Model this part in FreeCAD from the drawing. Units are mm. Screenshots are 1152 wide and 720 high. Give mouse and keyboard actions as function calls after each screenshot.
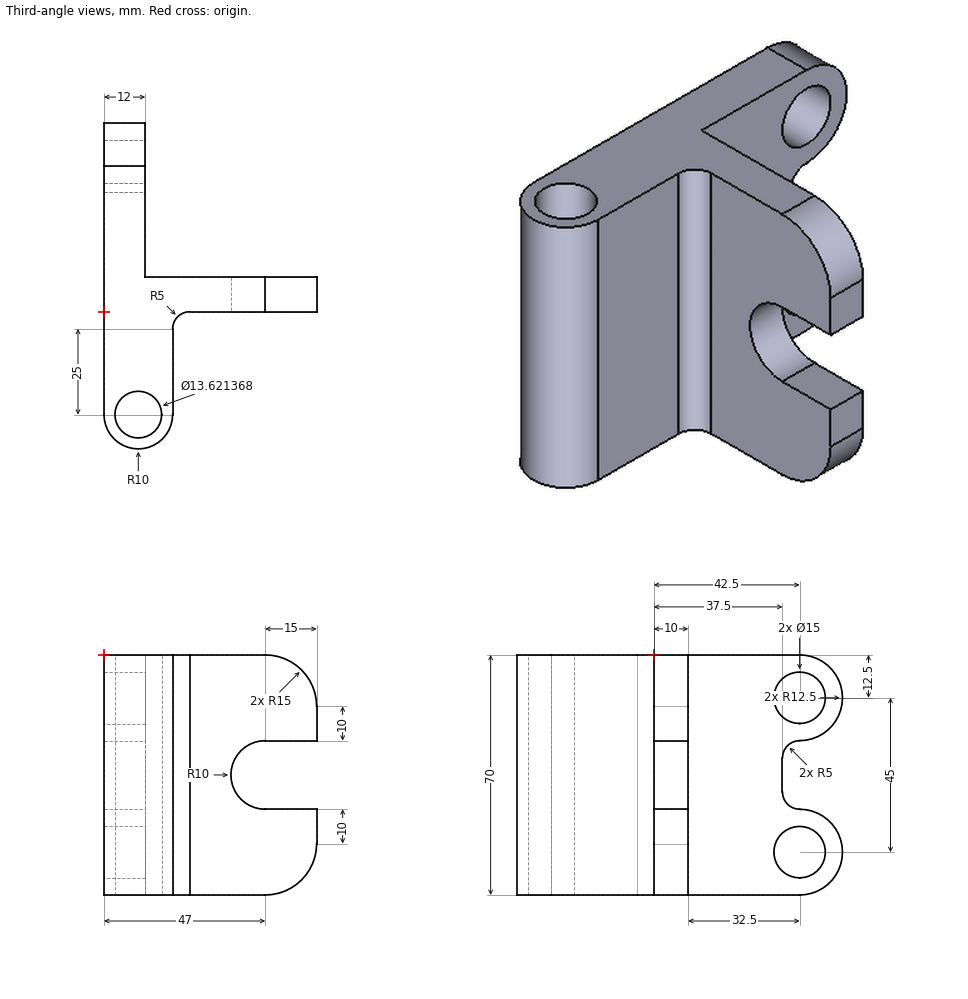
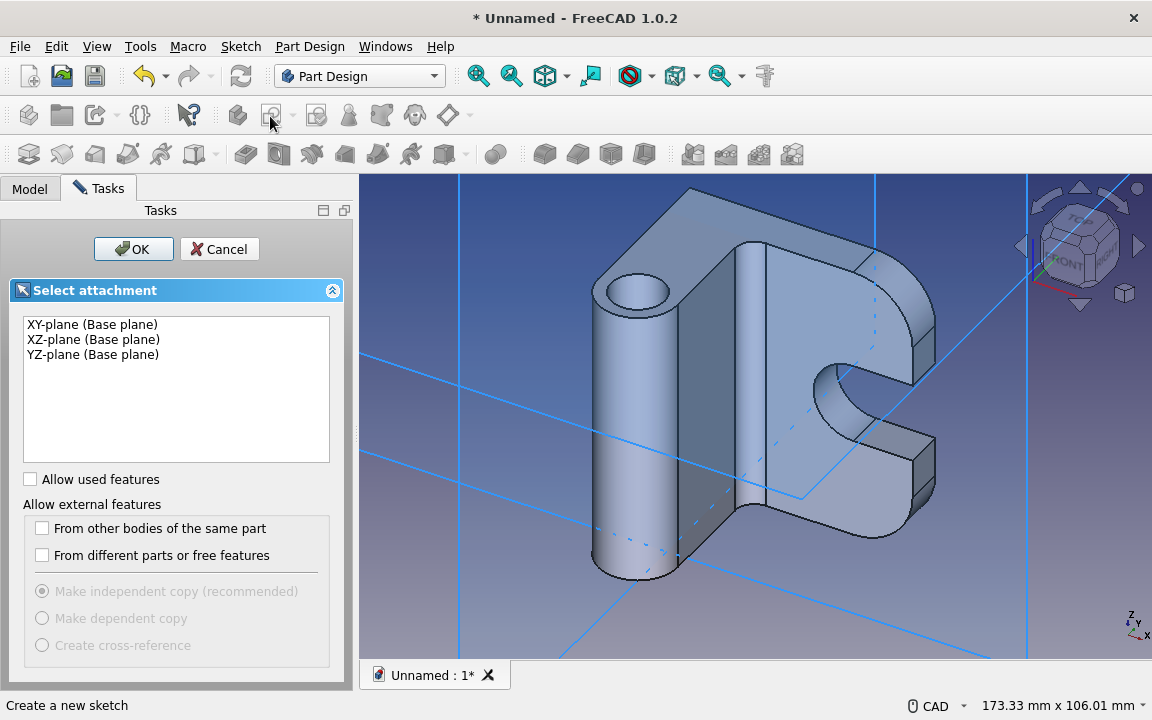
click(84, 354)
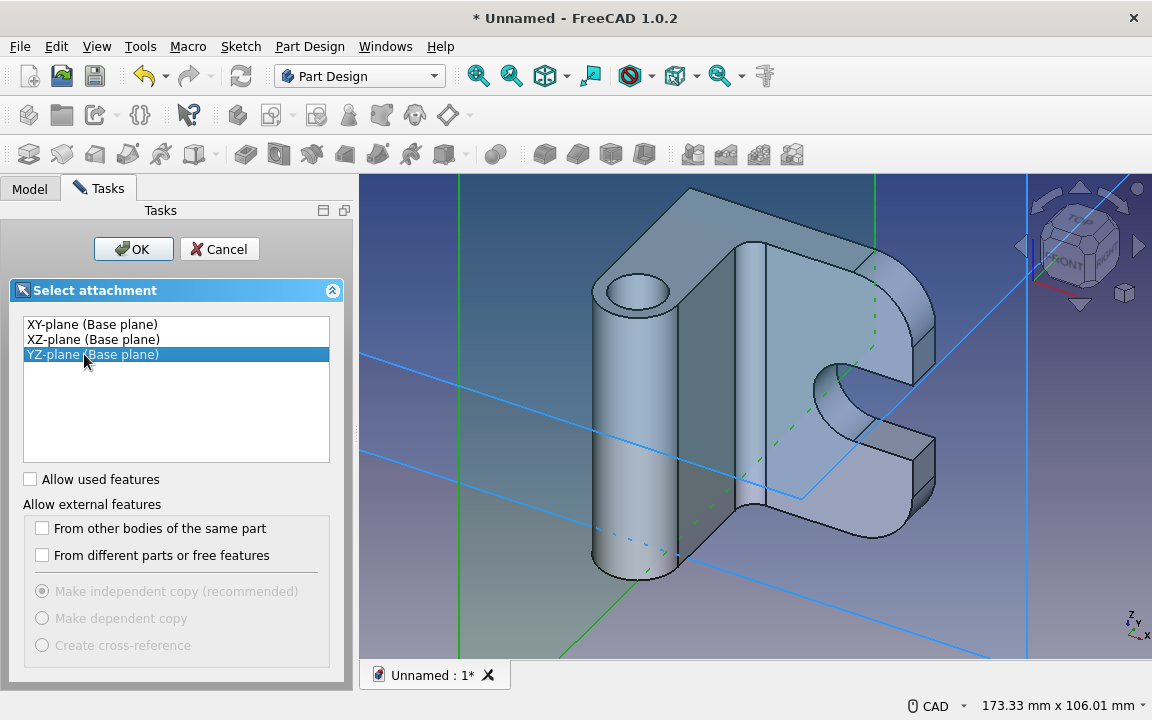
click(134, 249)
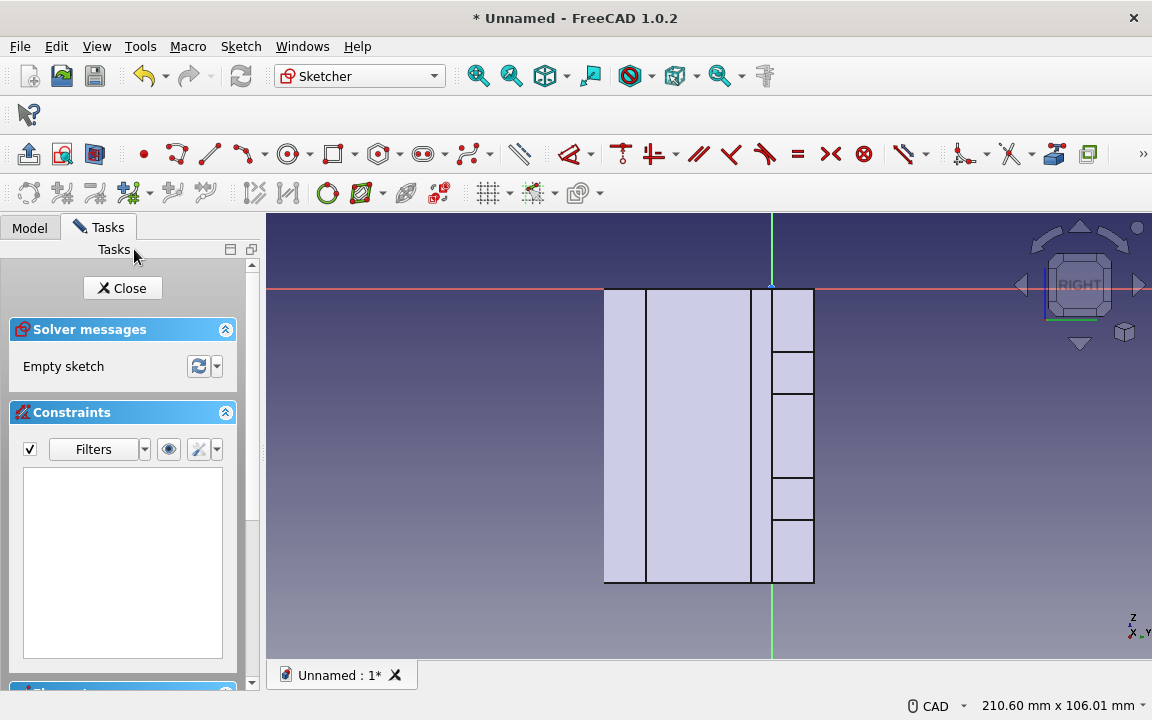
click(95, 154)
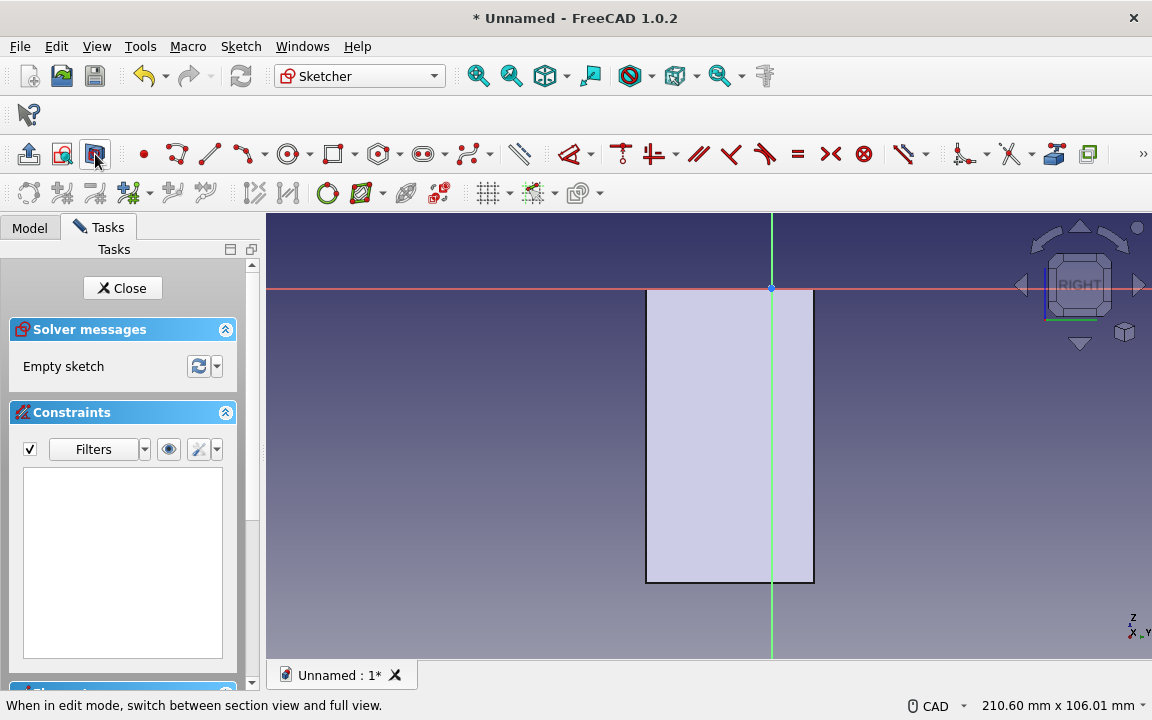
scroll(294, 436, down, 1)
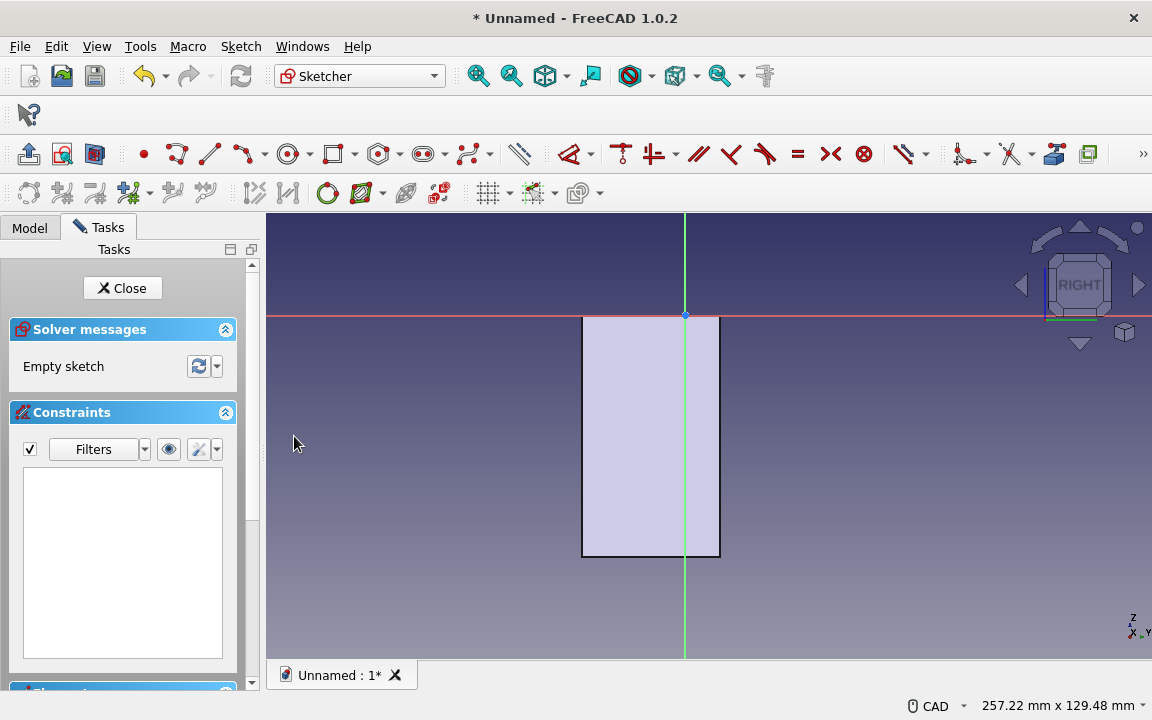
click(177, 154)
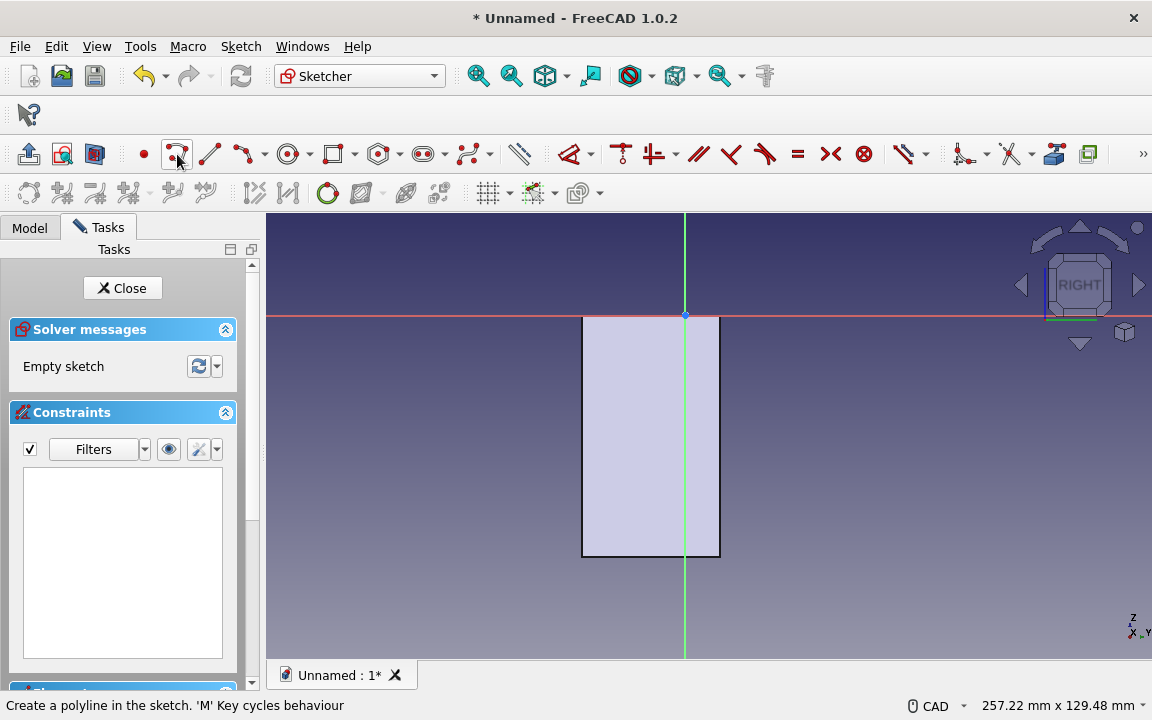
click(832, 557)
click(720, 557)
click(720, 316)
click(832, 325)
right_click(832, 325)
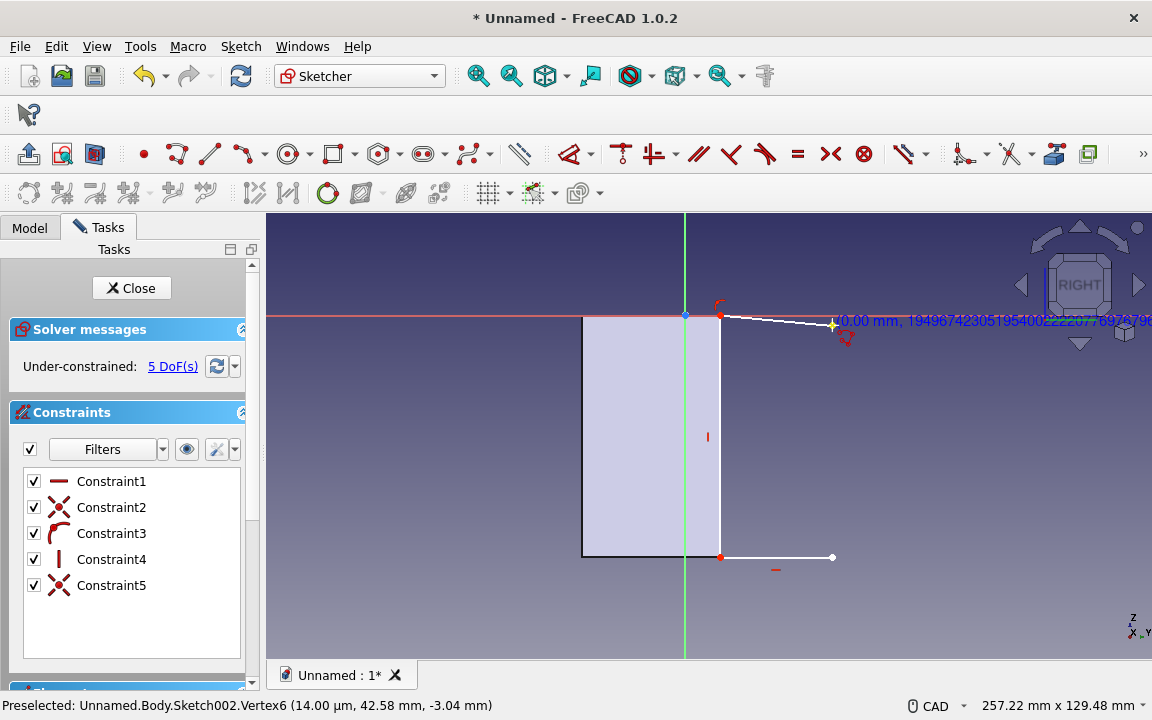
click(210, 154)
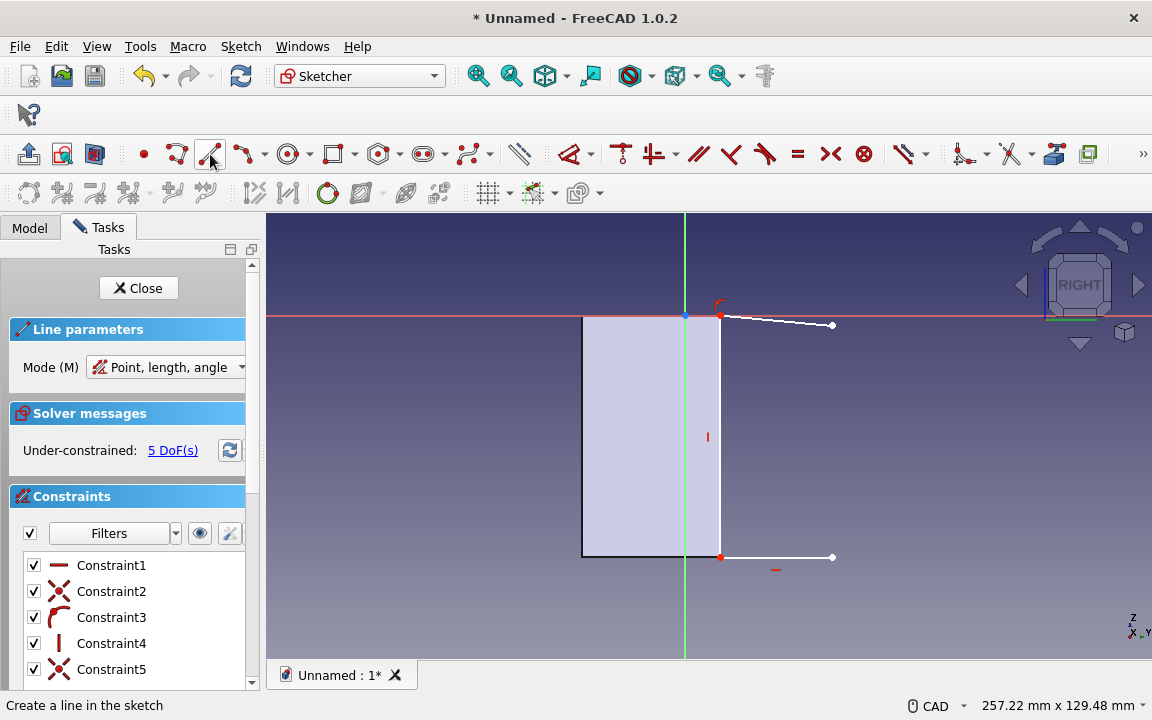
click(815, 419)
click(815, 453)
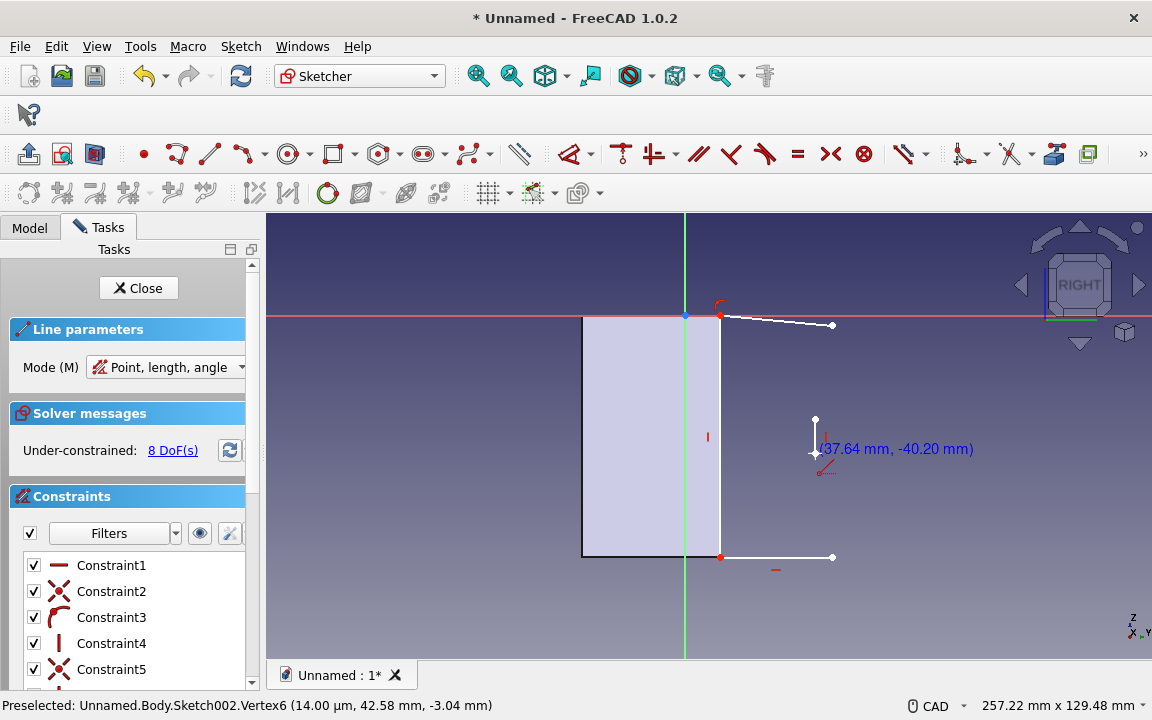
click(242, 154)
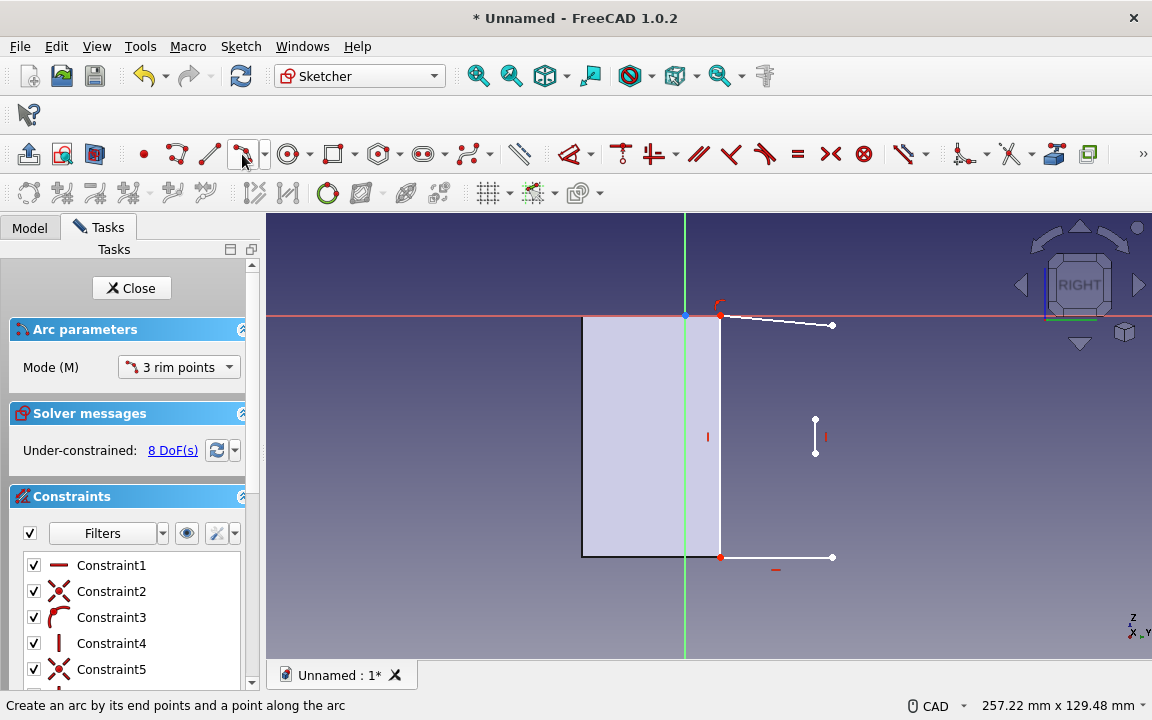
click(832, 326)
click(832, 402)
click(875, 359)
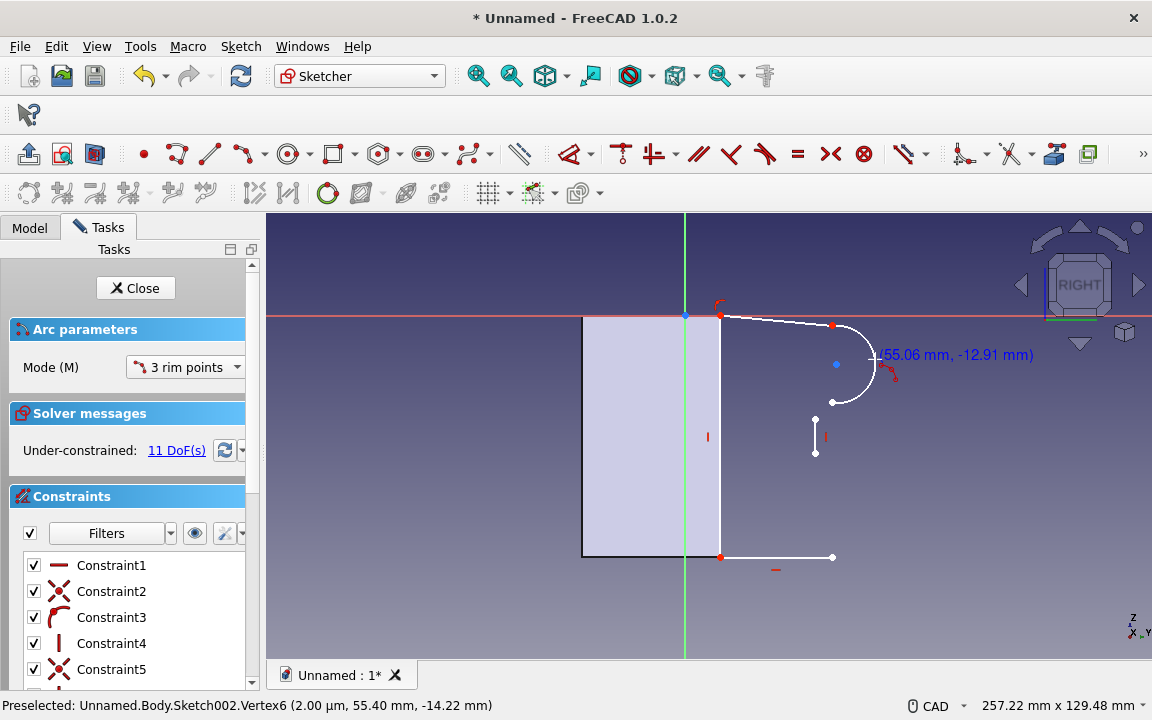
click(832, 403)
click(815, 420)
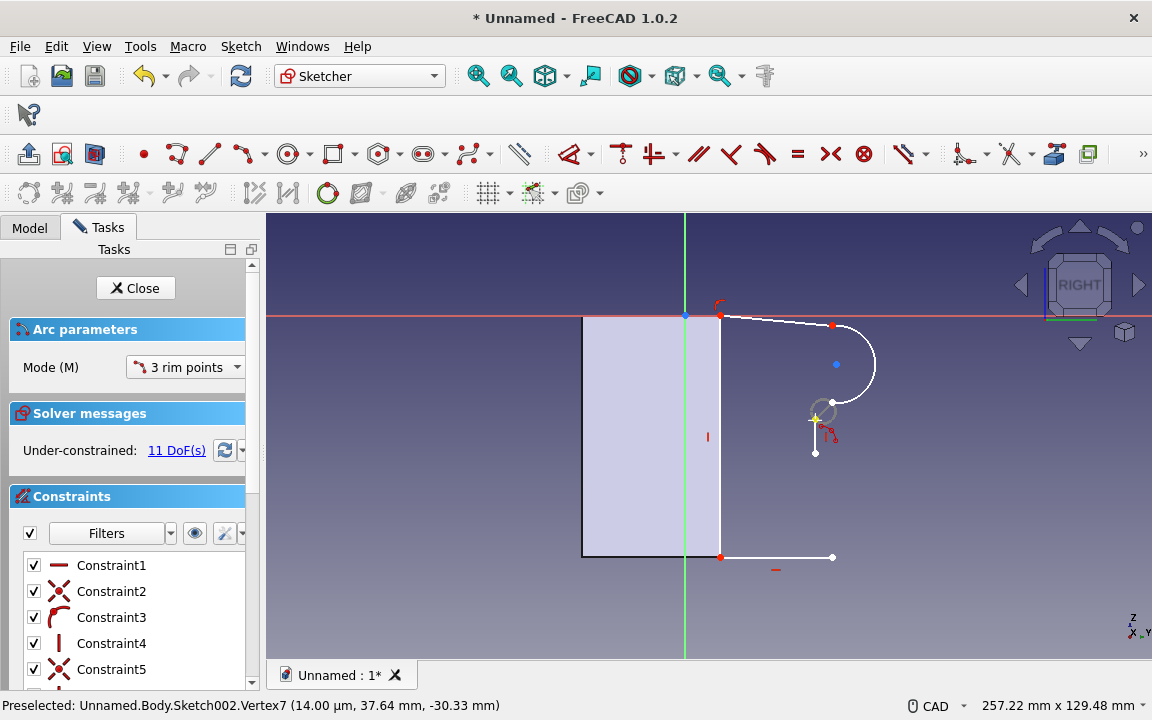
scroll(820, 407, up, 6)